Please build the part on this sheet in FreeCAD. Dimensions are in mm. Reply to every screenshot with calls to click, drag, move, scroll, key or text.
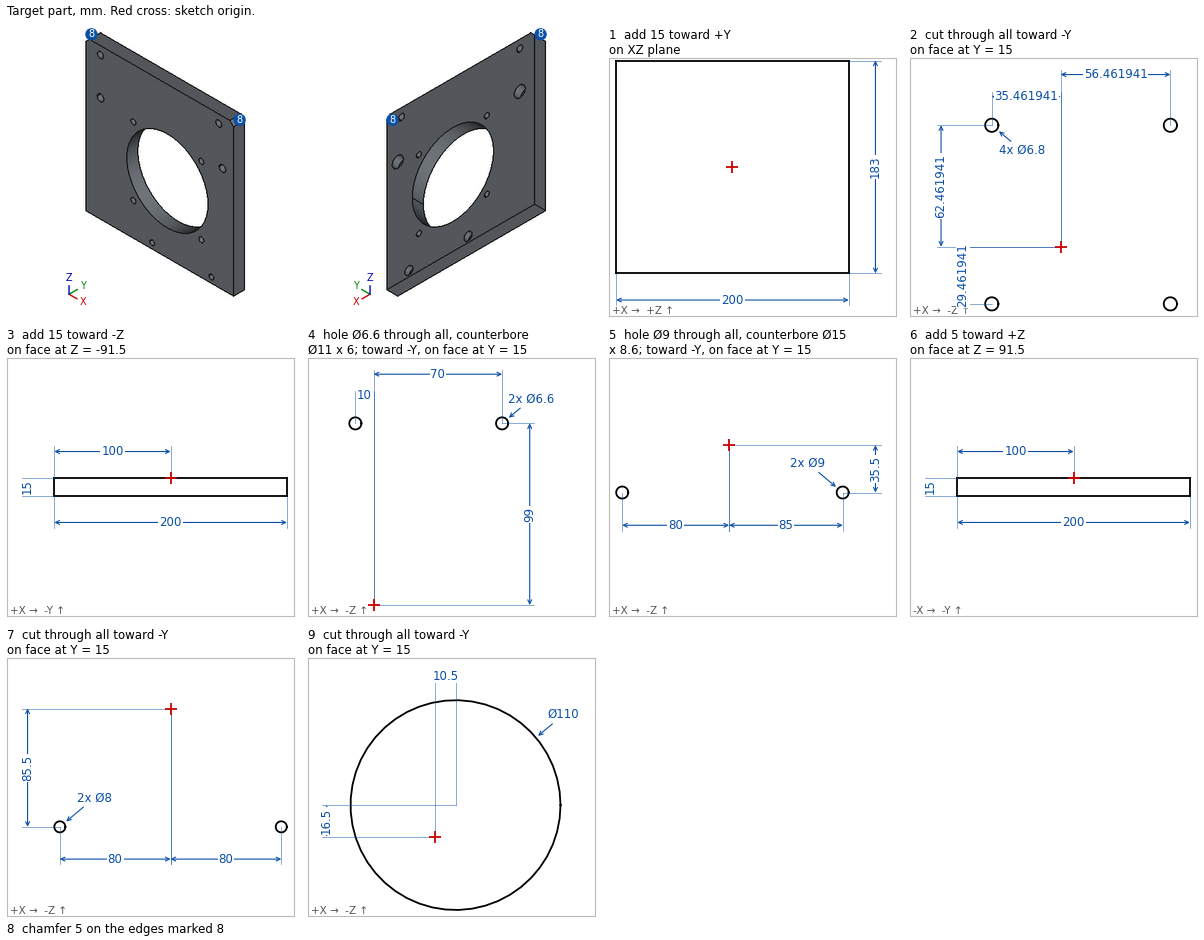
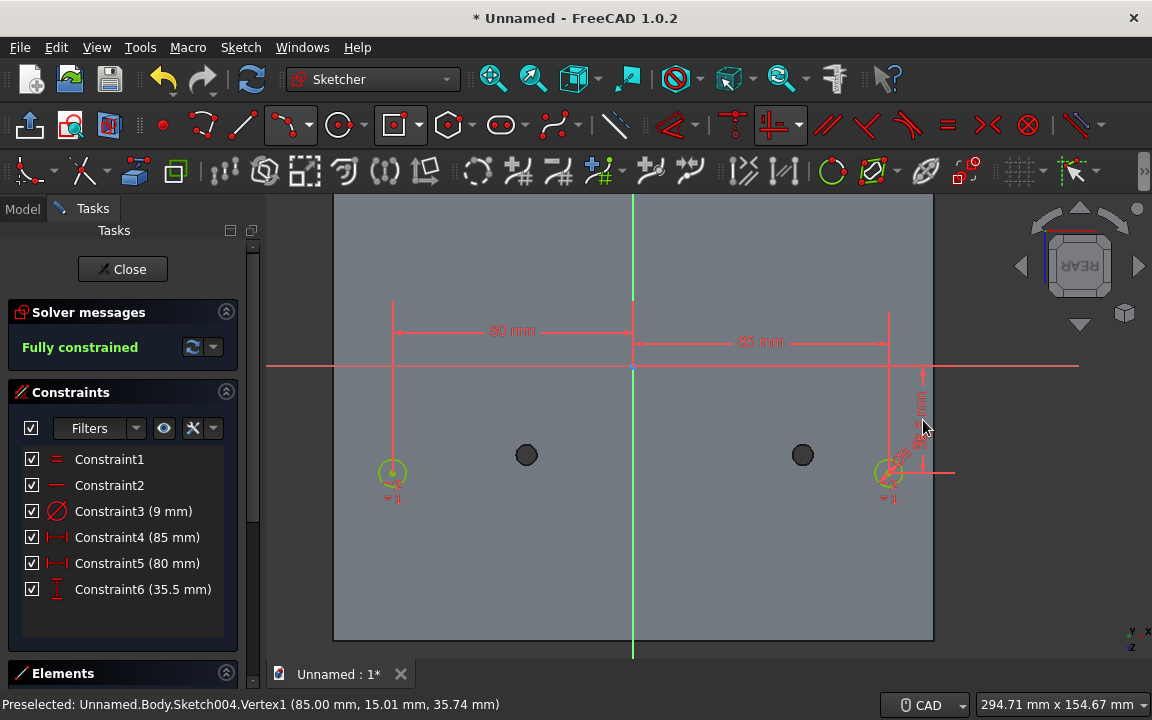
click(123, 269)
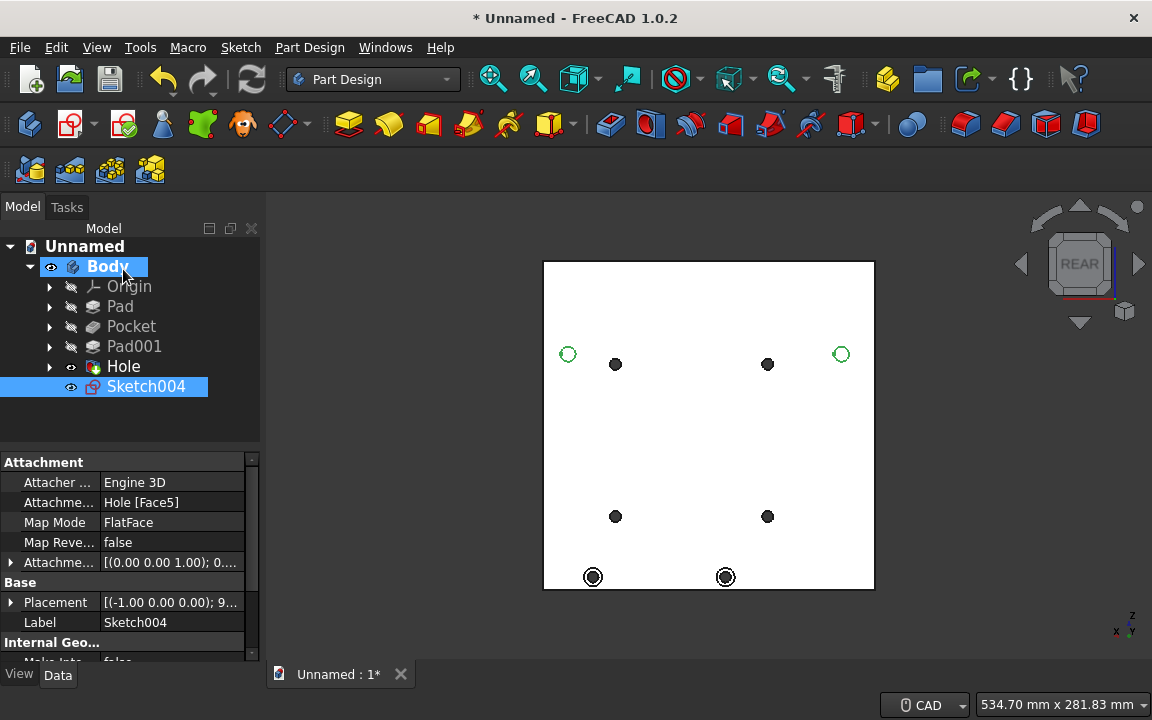
click(652, 124)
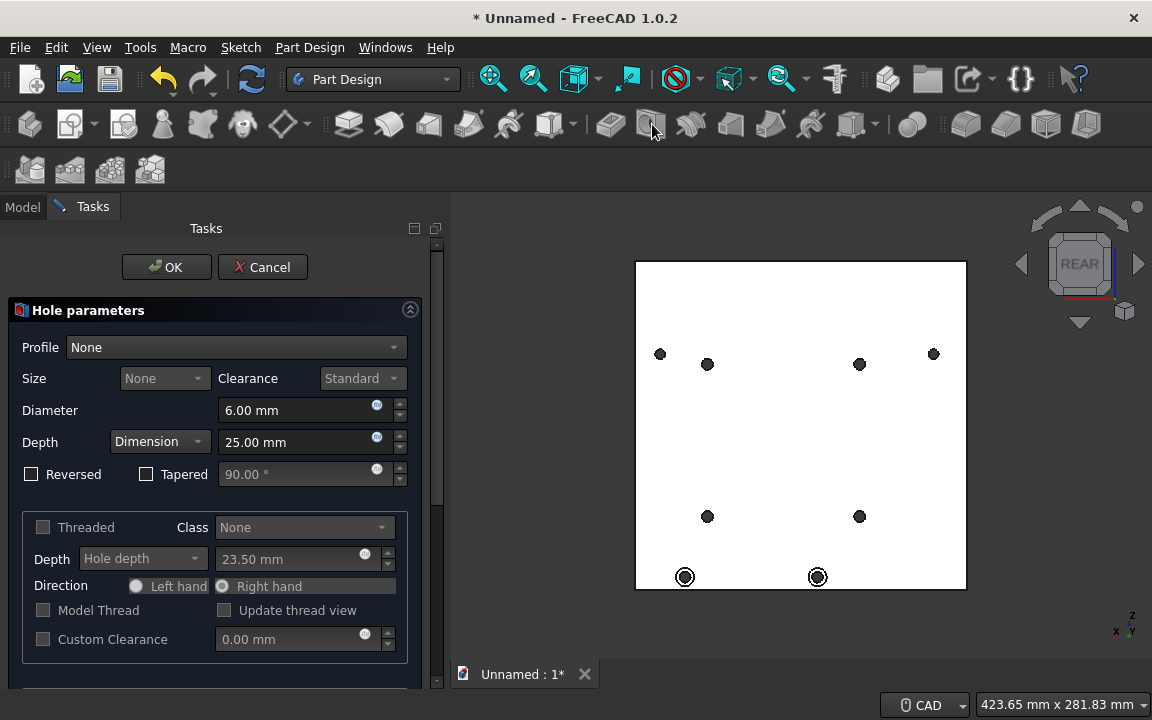
triple_click(305, 410)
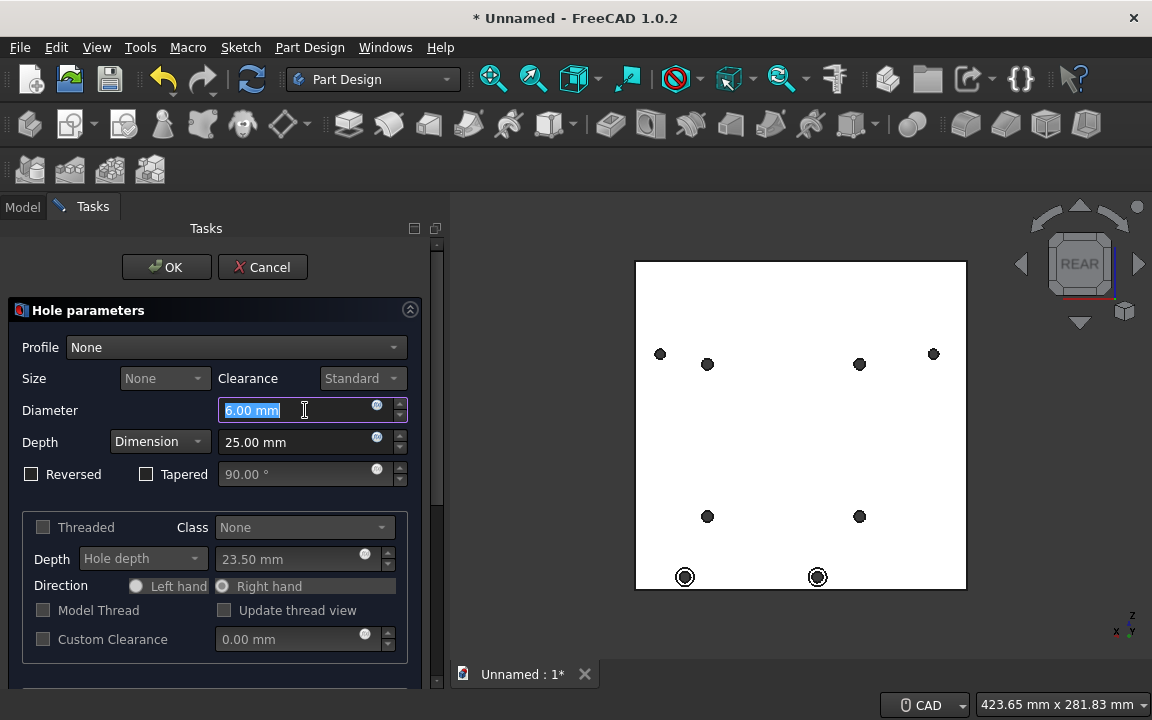
text(9)
key(Tab)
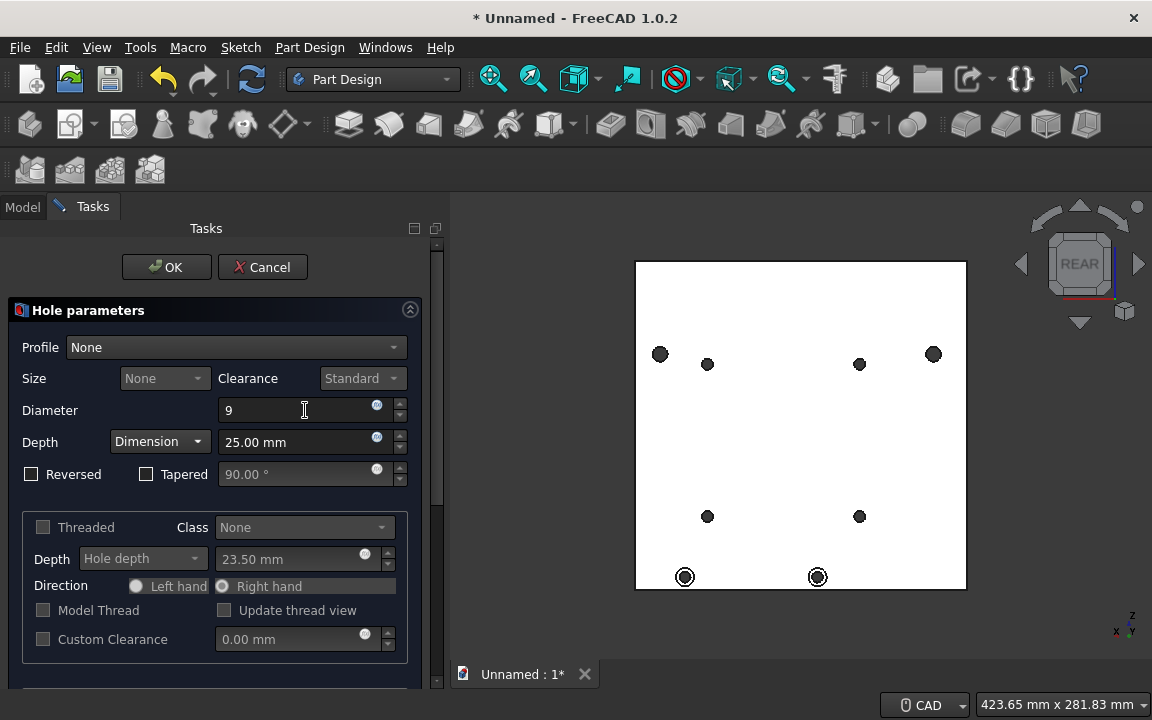
click(161, 442)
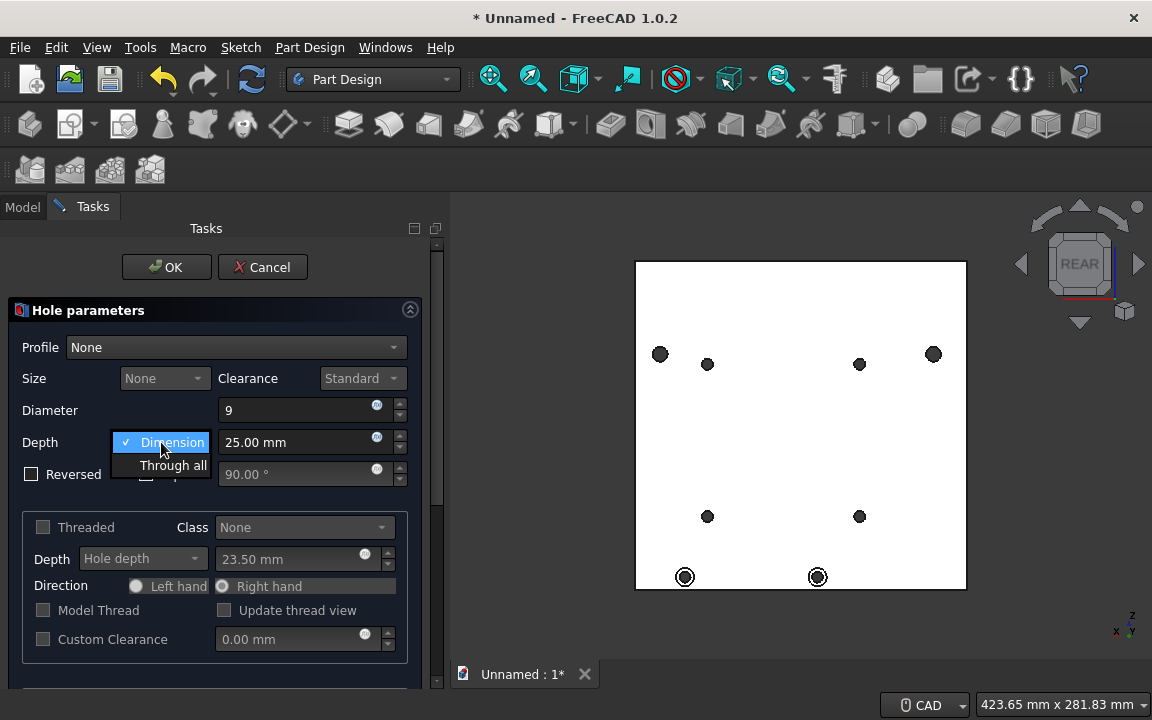
click(160, 466)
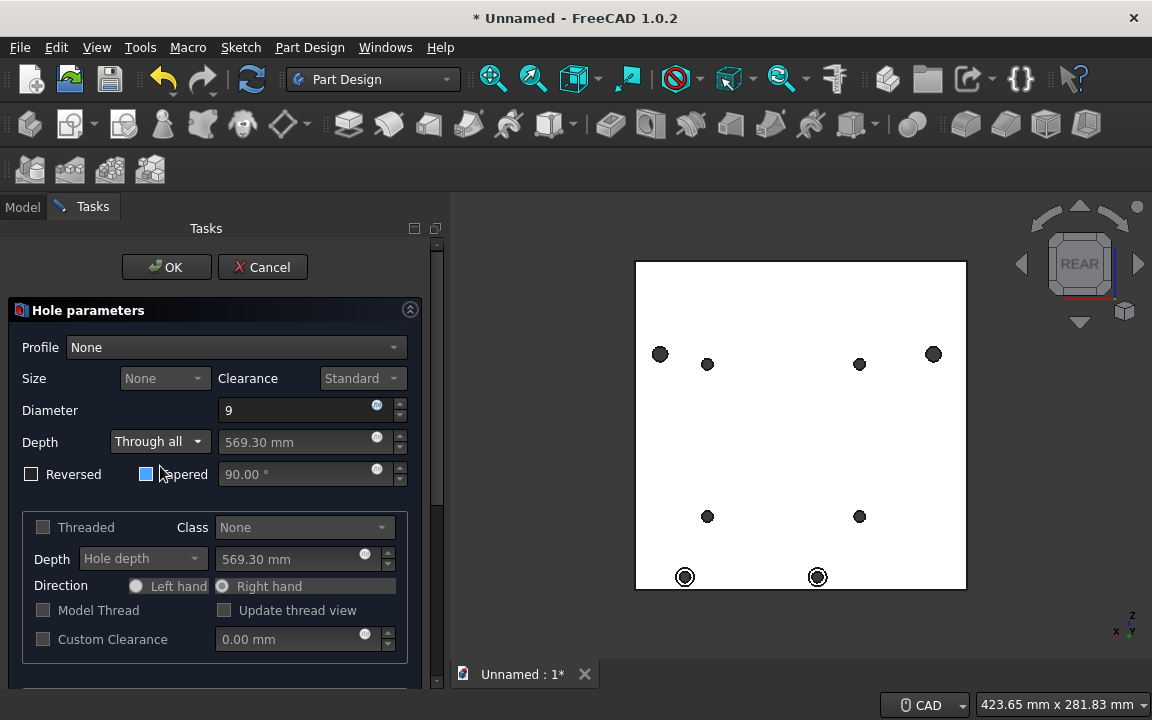
scroll(437, 463, down, 2)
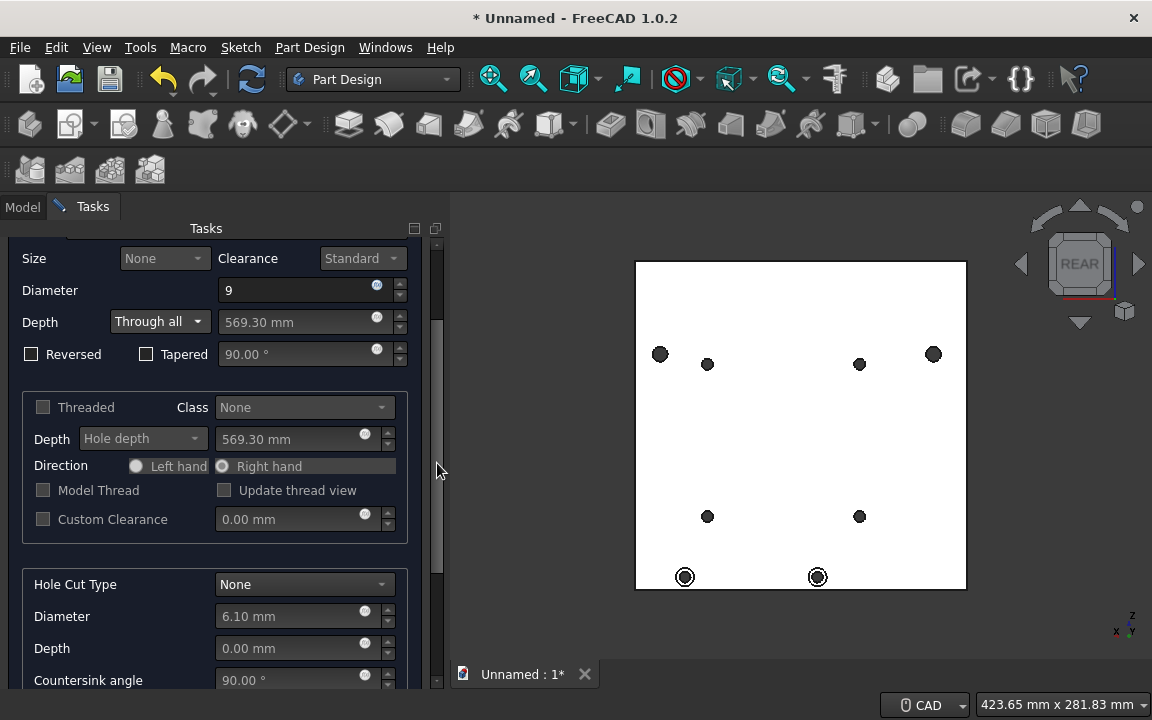
click(306, 584)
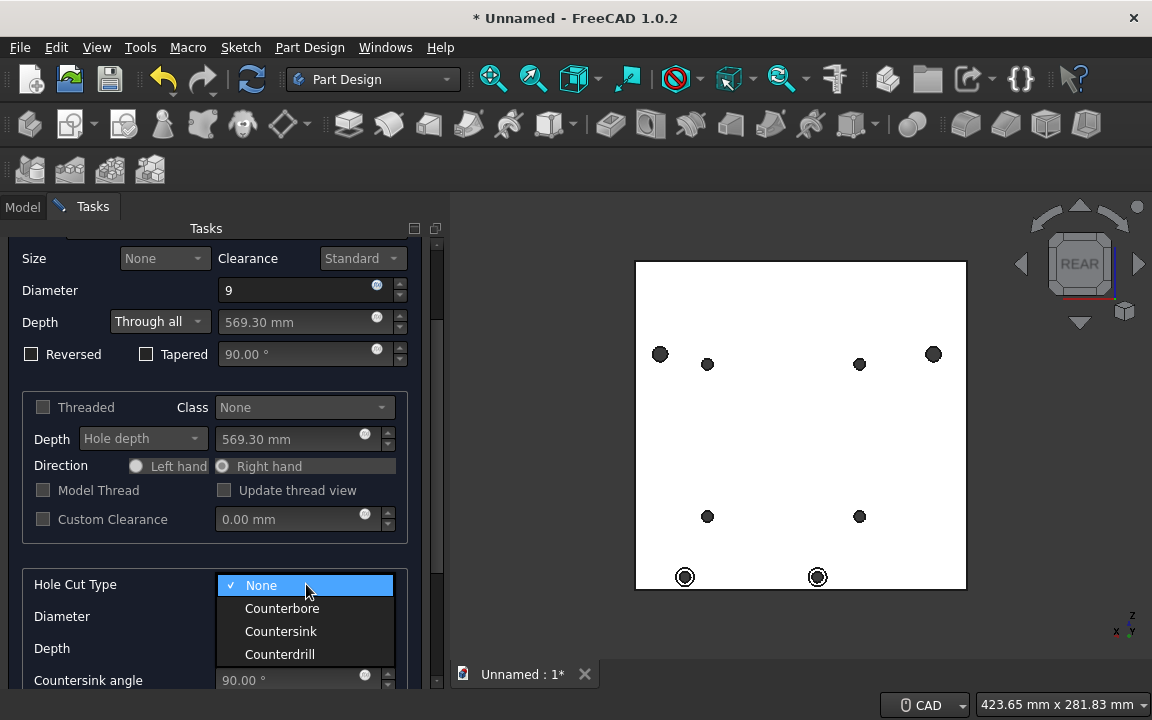
click(304, 608)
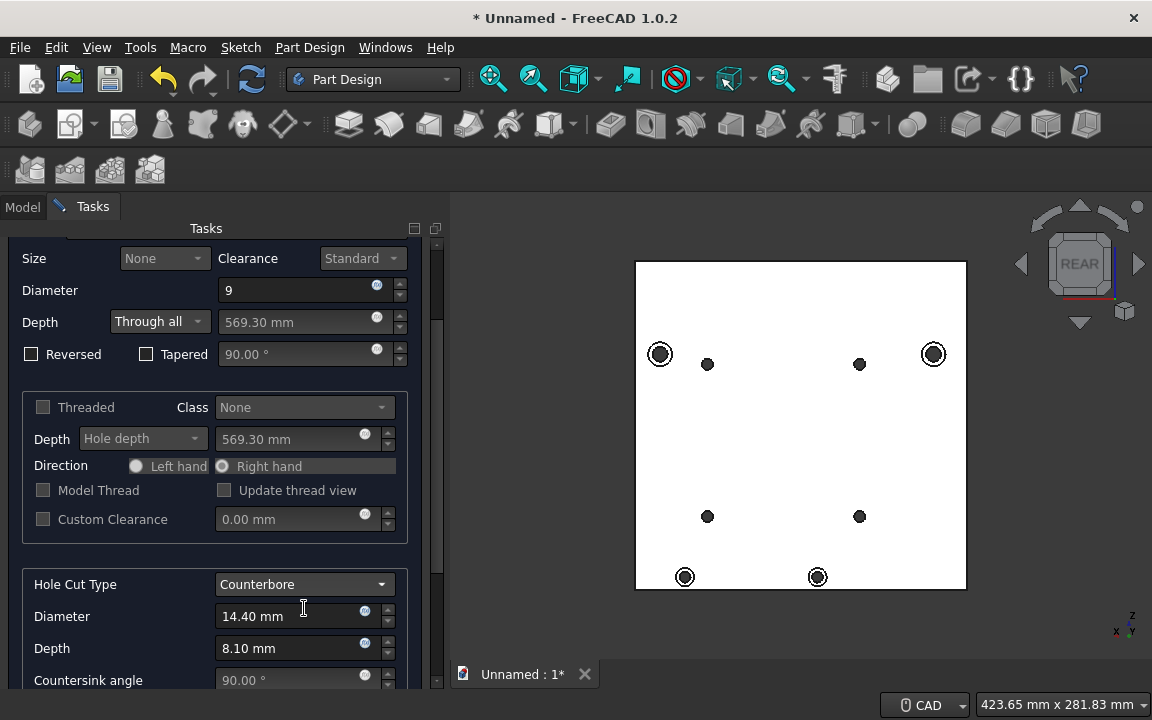
triple_click(298, 616)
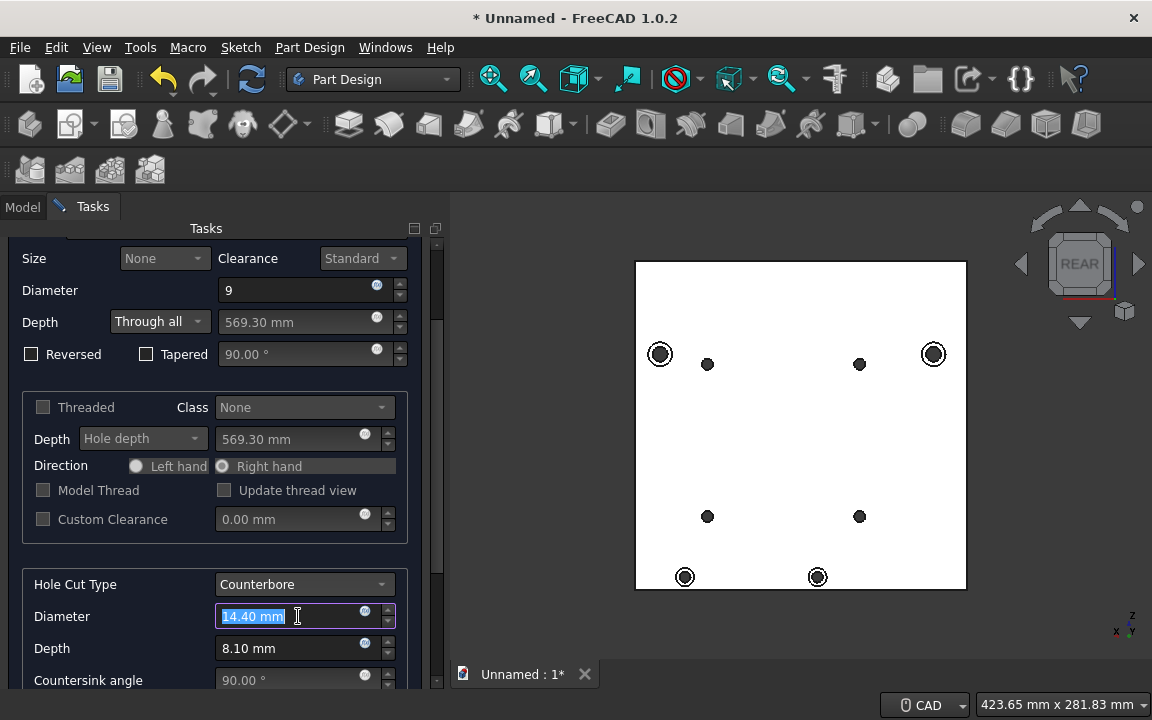
text(15)
key(Tab)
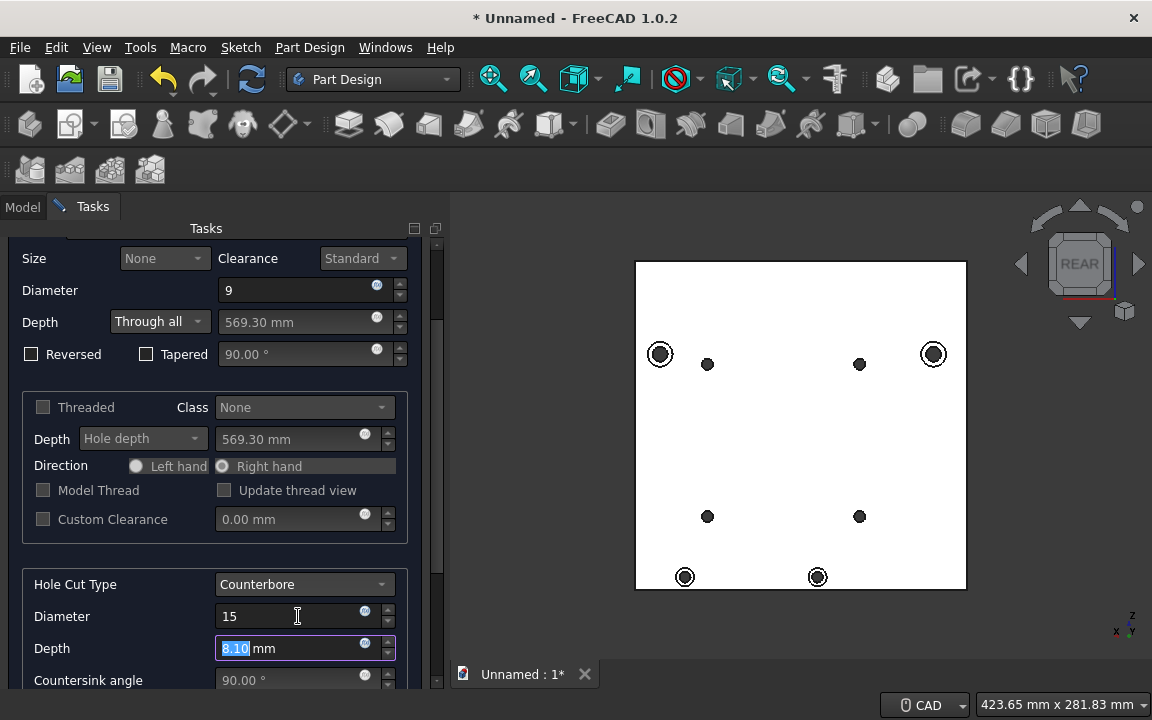
text(8.6)
key(Tab)